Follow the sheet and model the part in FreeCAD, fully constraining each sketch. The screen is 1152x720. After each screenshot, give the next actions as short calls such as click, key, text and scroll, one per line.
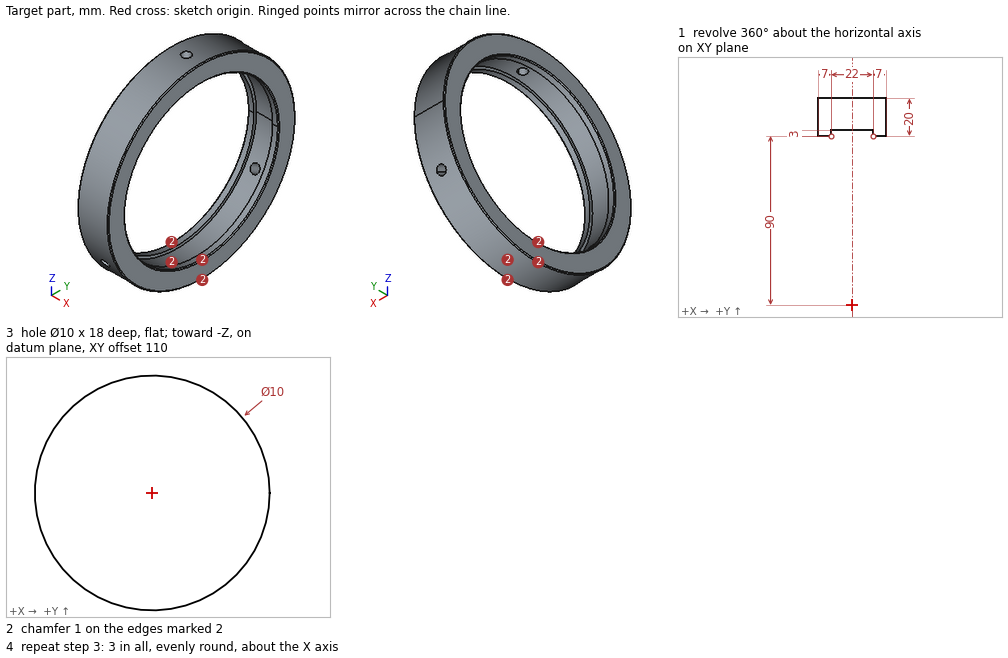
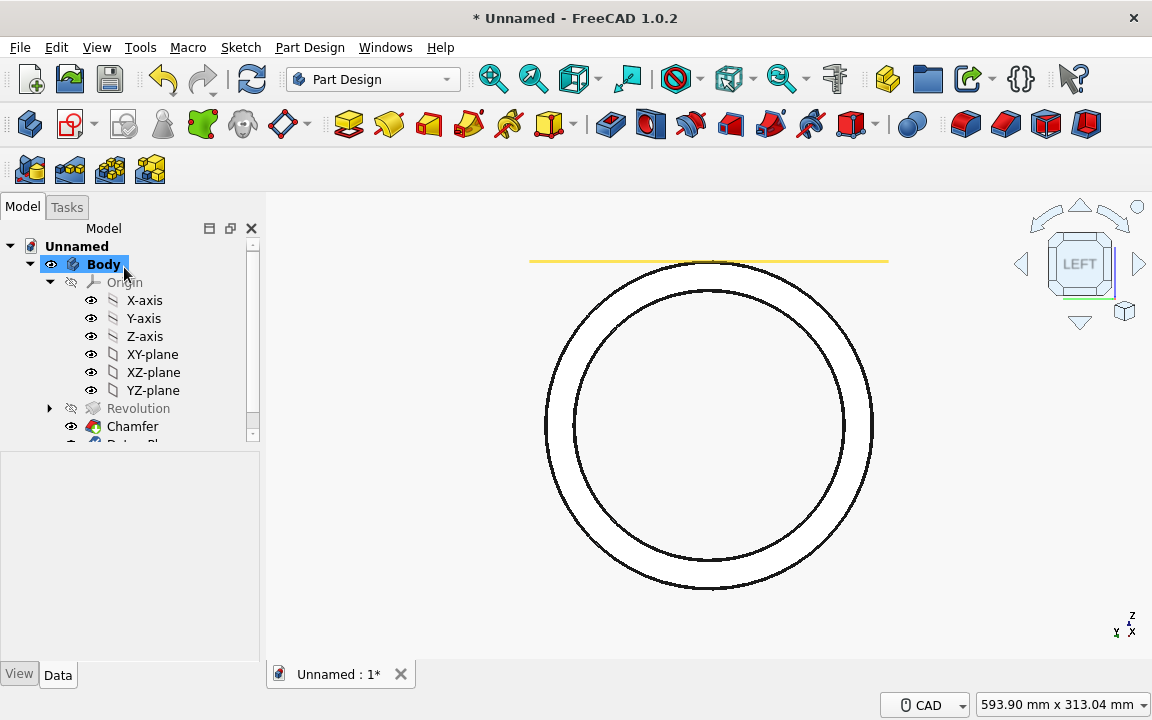
scroll(100, 332, down, 3)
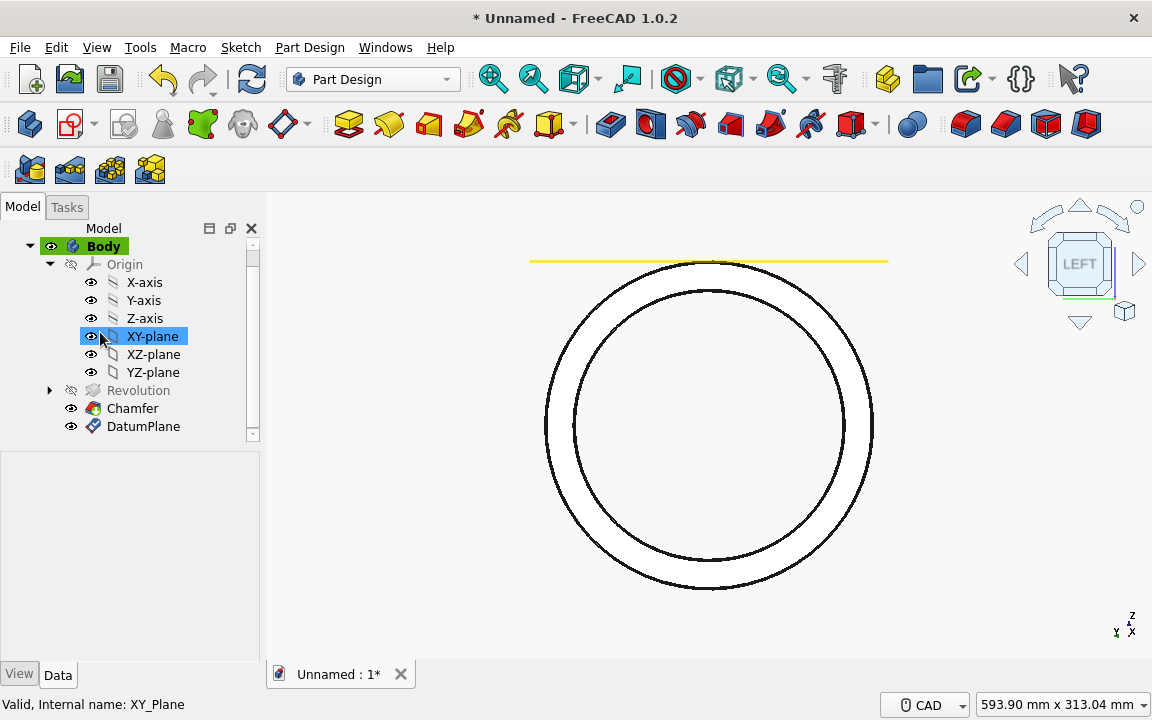
click(116, 426)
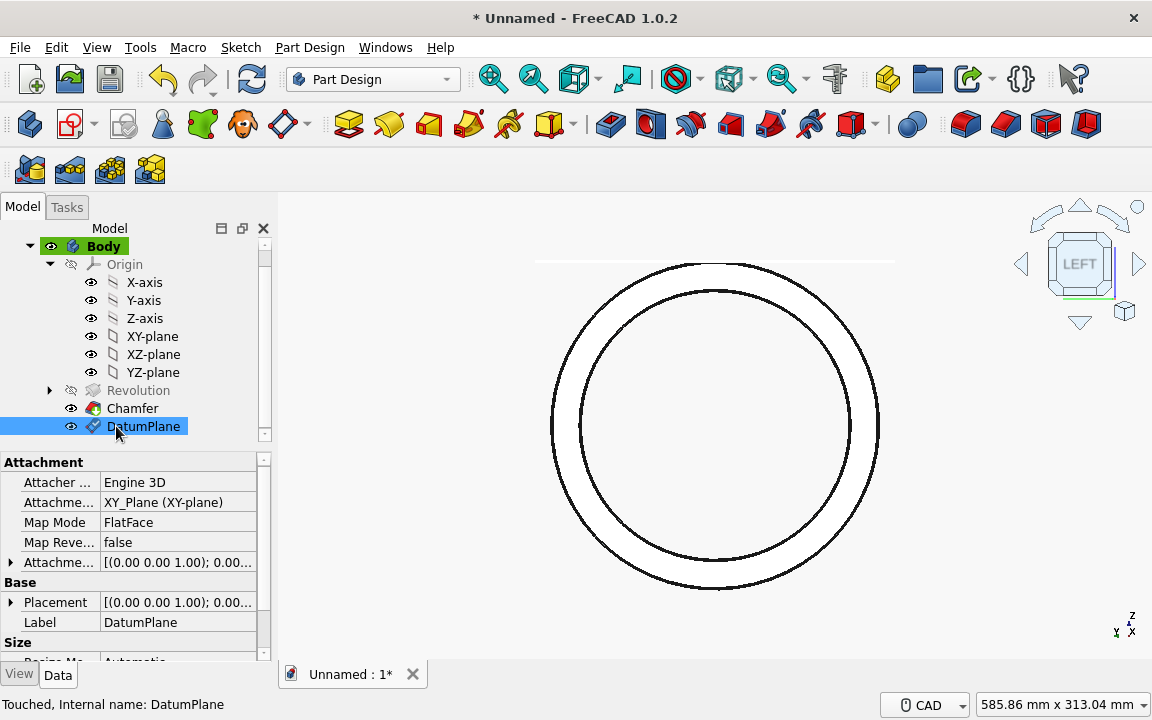
click(70, 124)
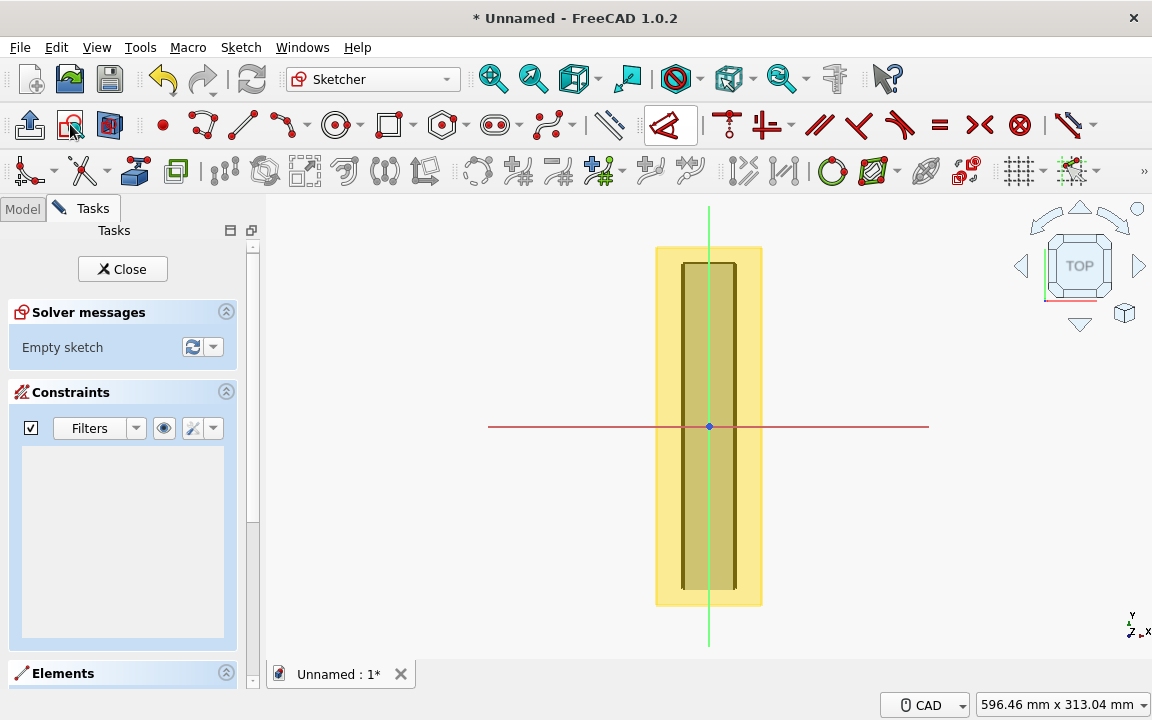
scroll(713, 427, up, 15)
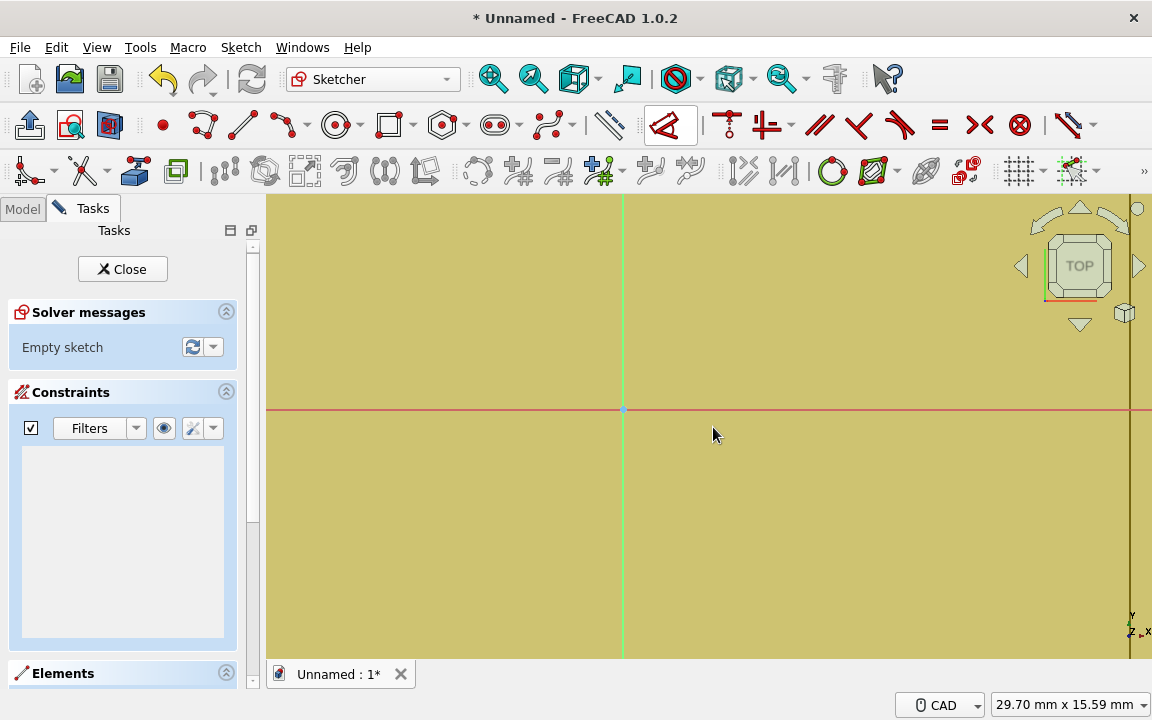
click(336, 126)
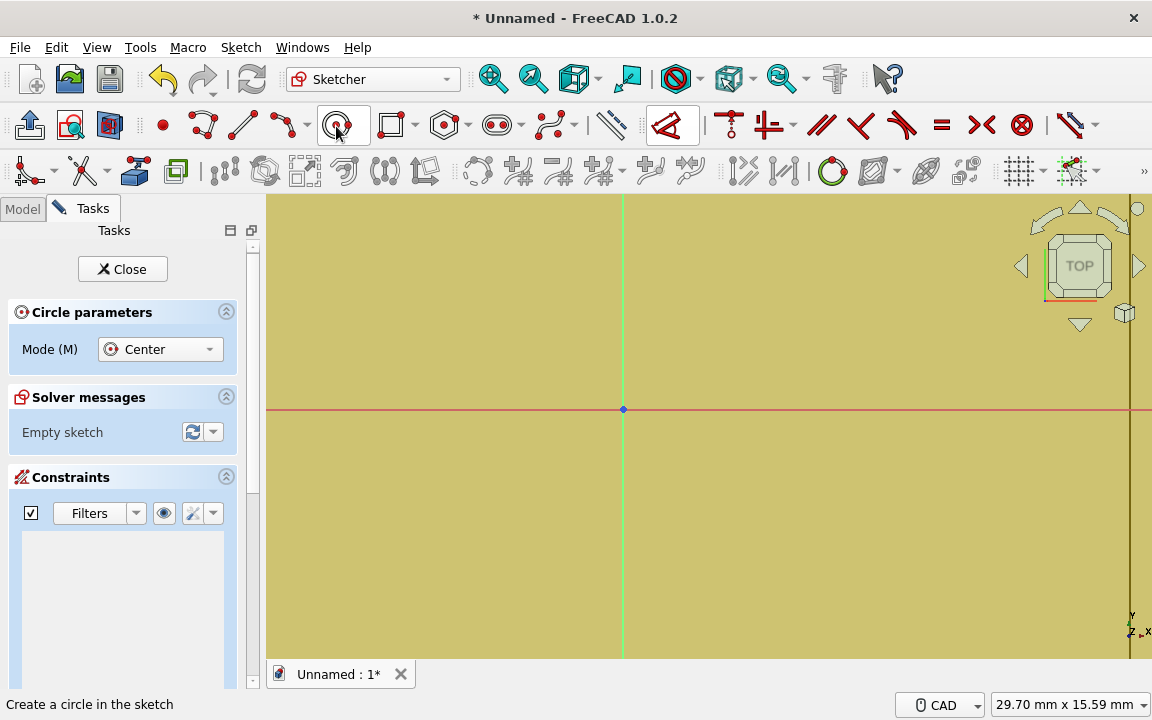
click(623, 410)
move(729, 304)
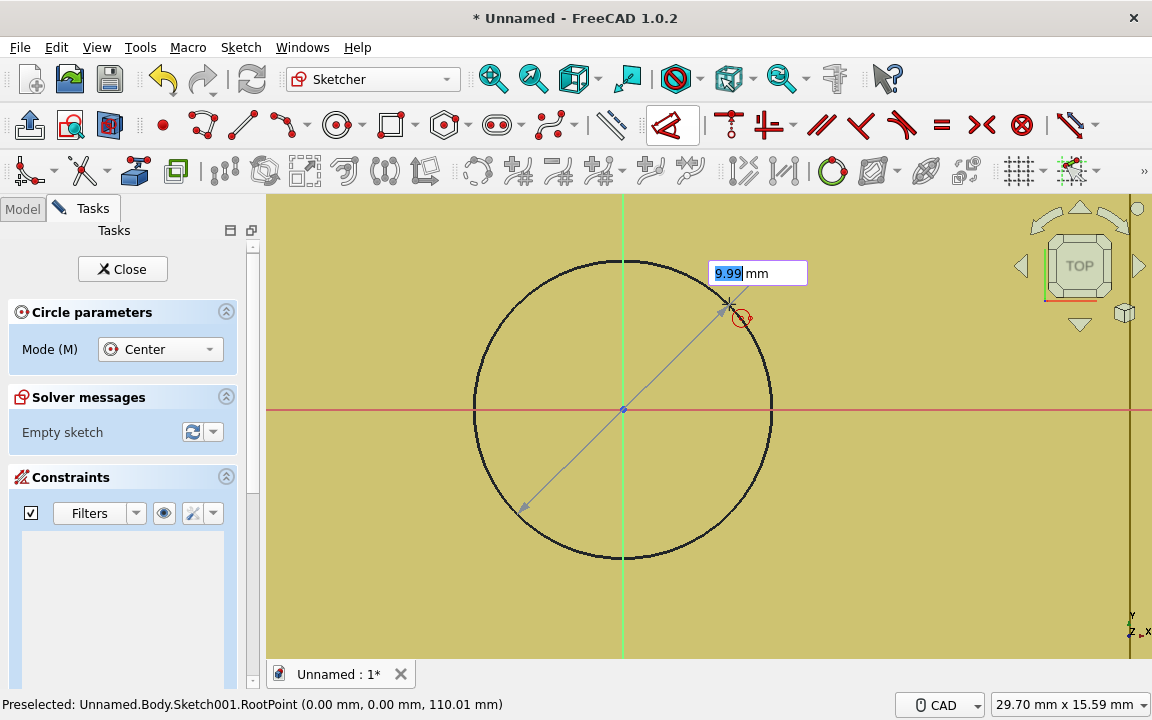
text(10)
key(Return)
key(Escape)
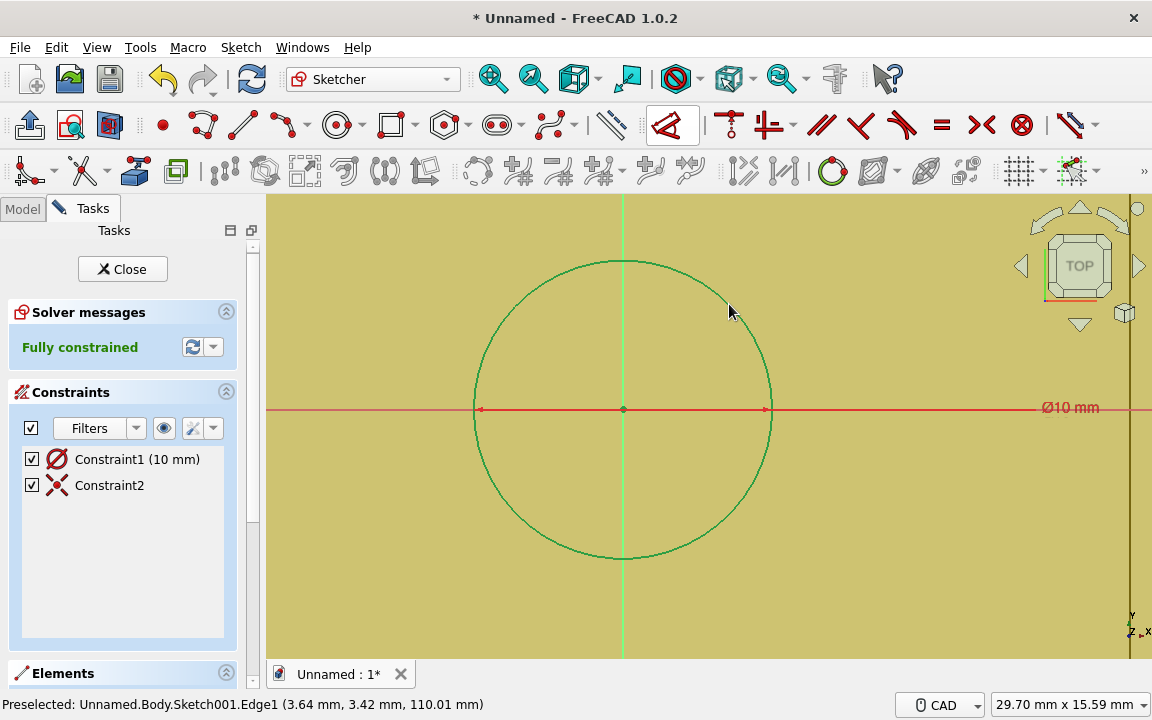
click(123, 269)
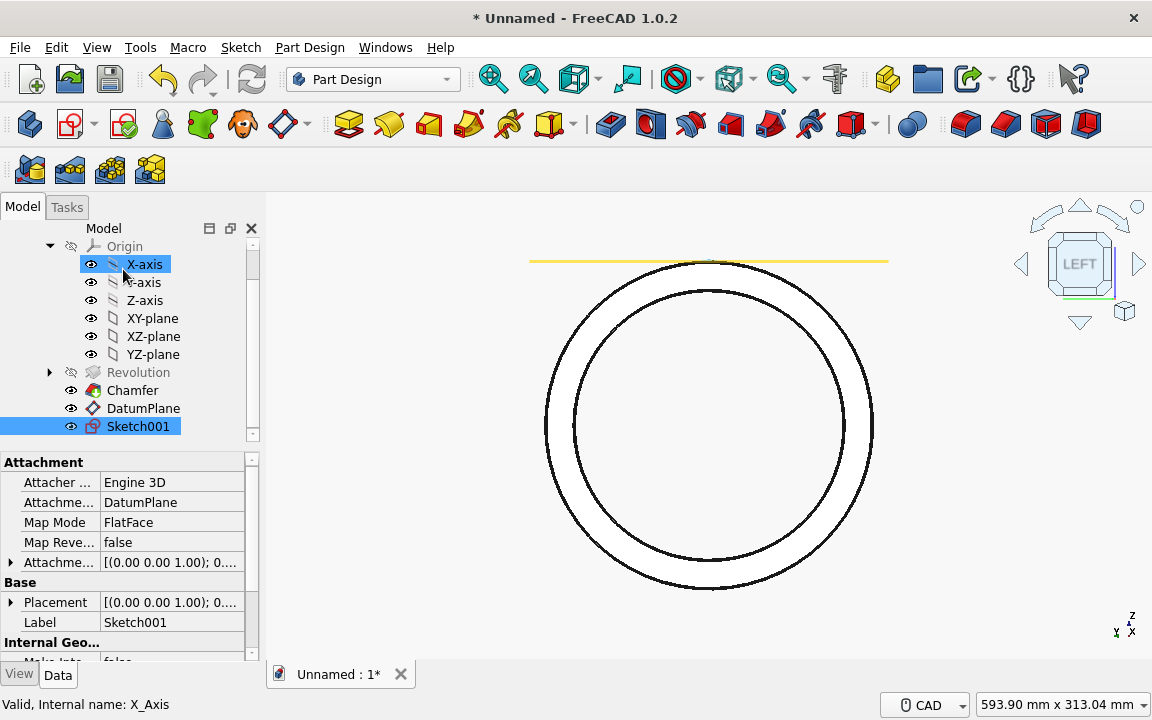
click(652, 124)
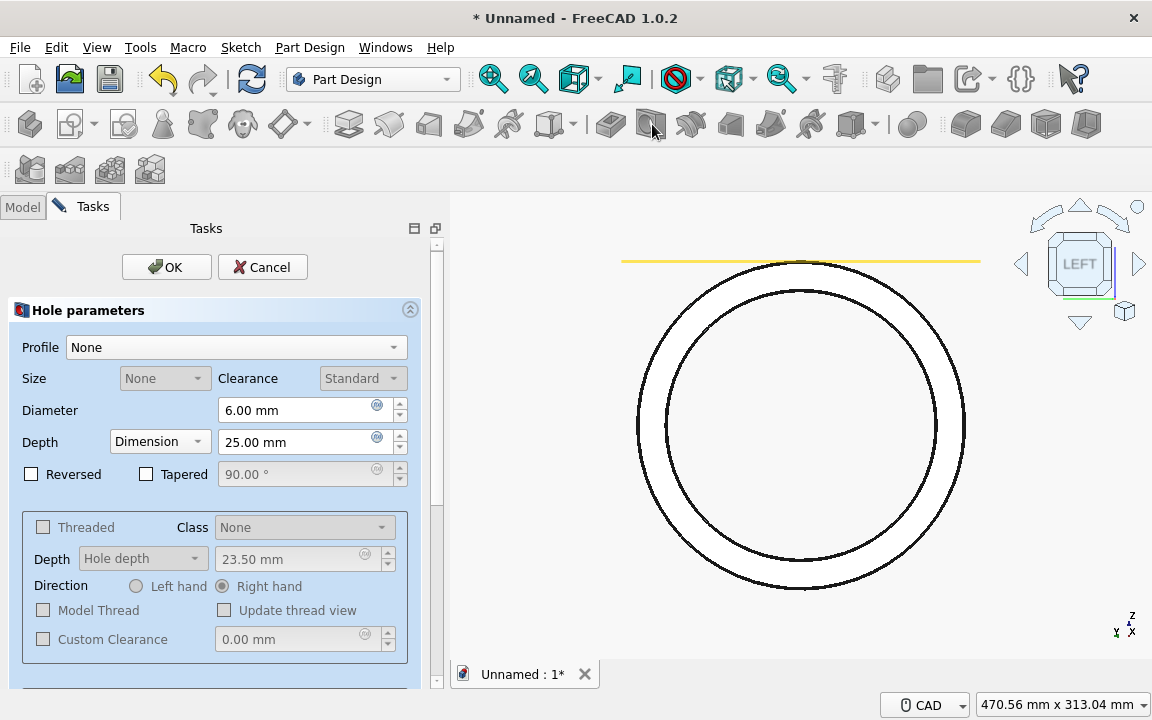
triple_click(305, 410)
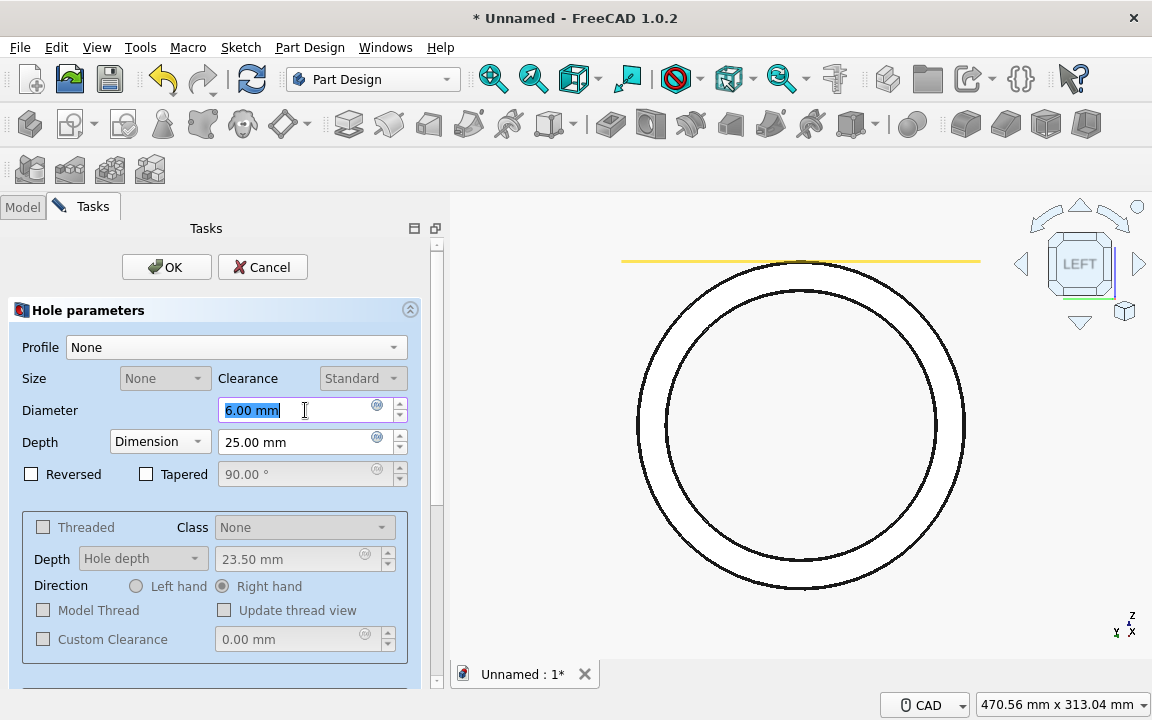
text(10)
key(Tab)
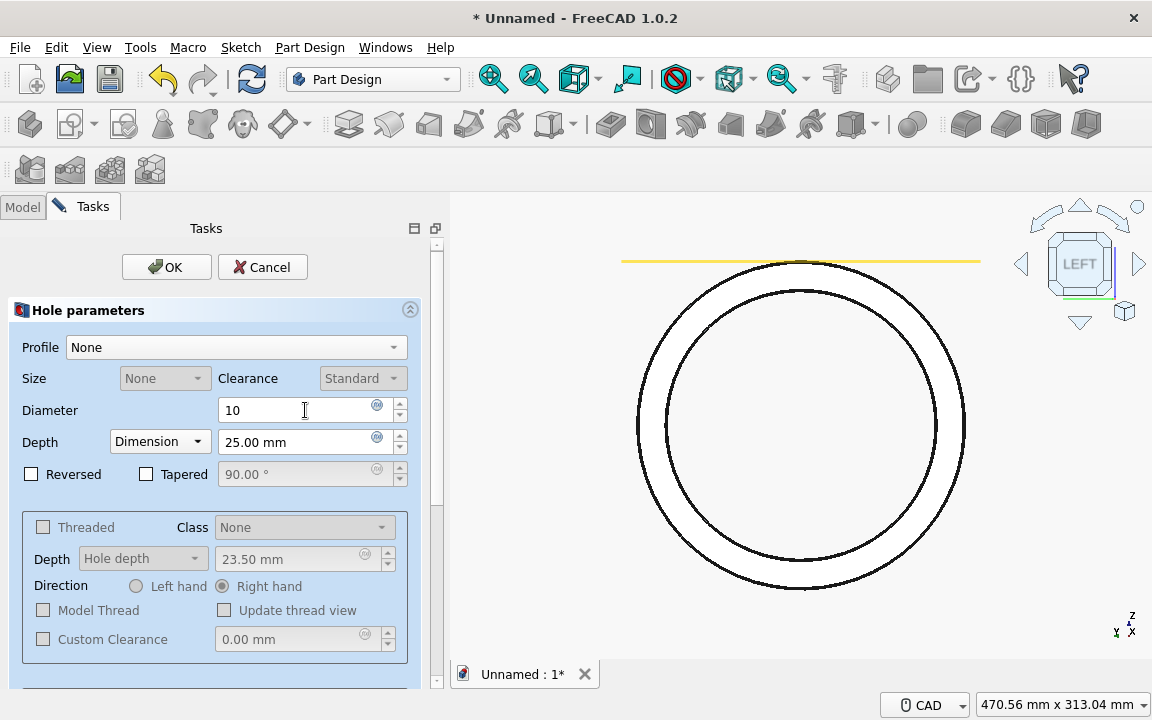
triple_click(305, 442)